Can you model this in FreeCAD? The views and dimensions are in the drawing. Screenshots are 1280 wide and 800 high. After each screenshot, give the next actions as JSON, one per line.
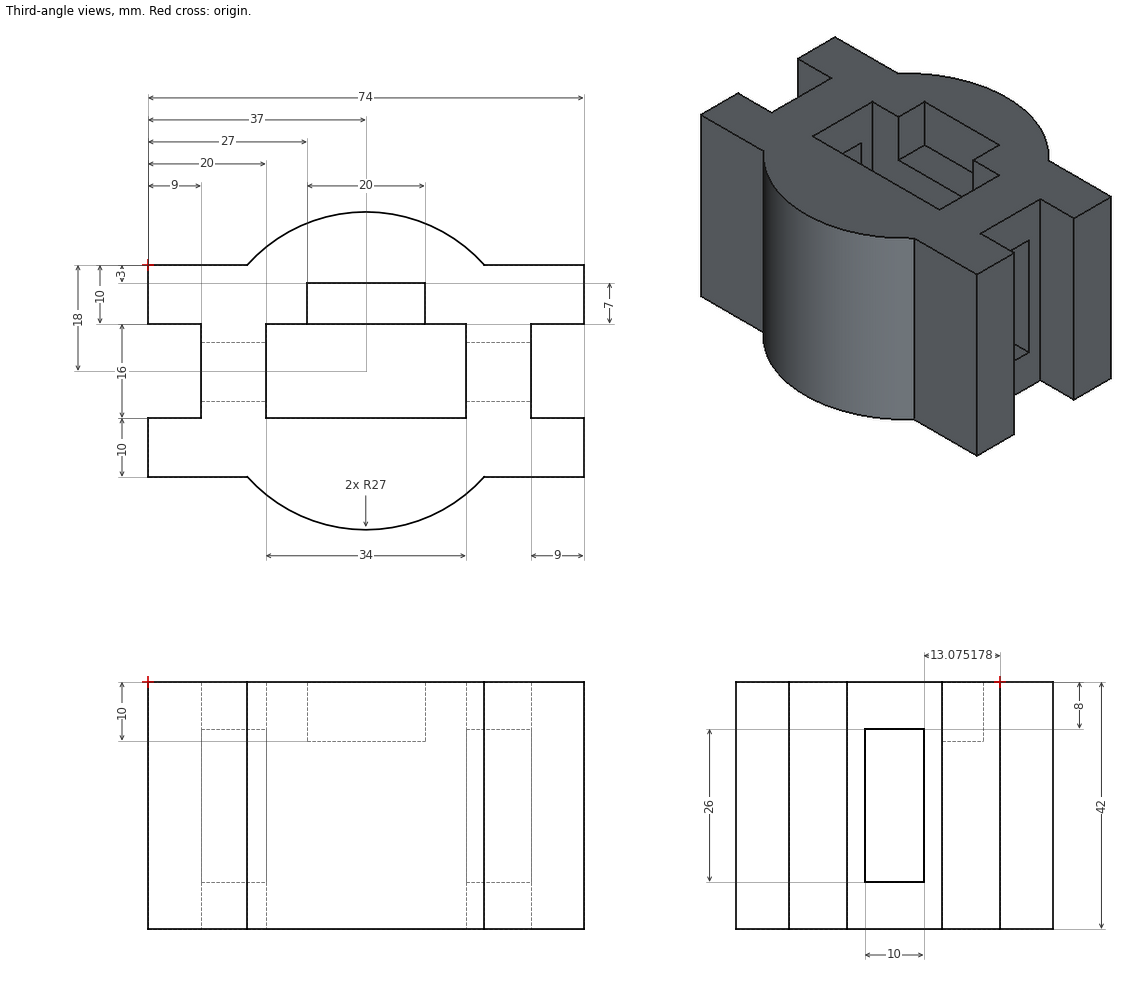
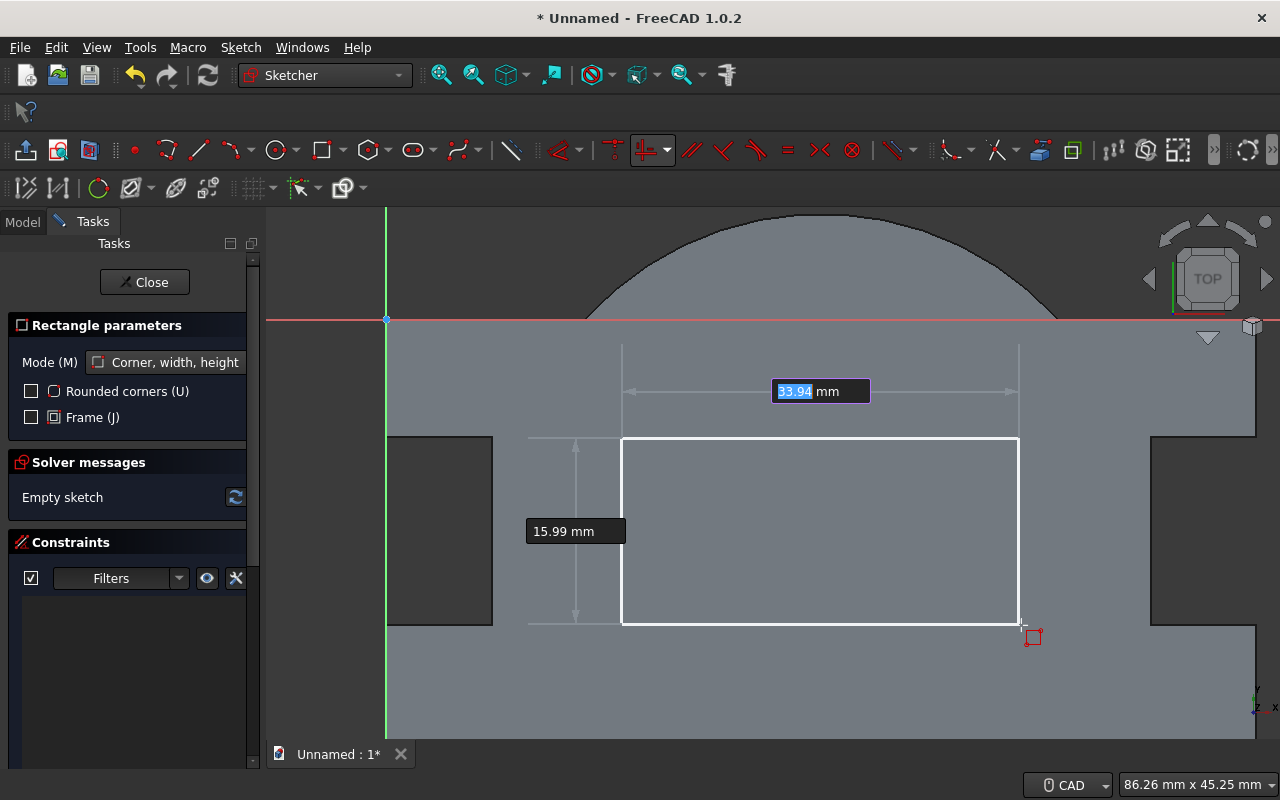
{"action": "type", "text": "34"}
{"action": "key", "text": "Tab"}
{"action": "type", "text": "16"}
{"action": "key", "text": "Return"}
{"action": "key", "text": "Escape"}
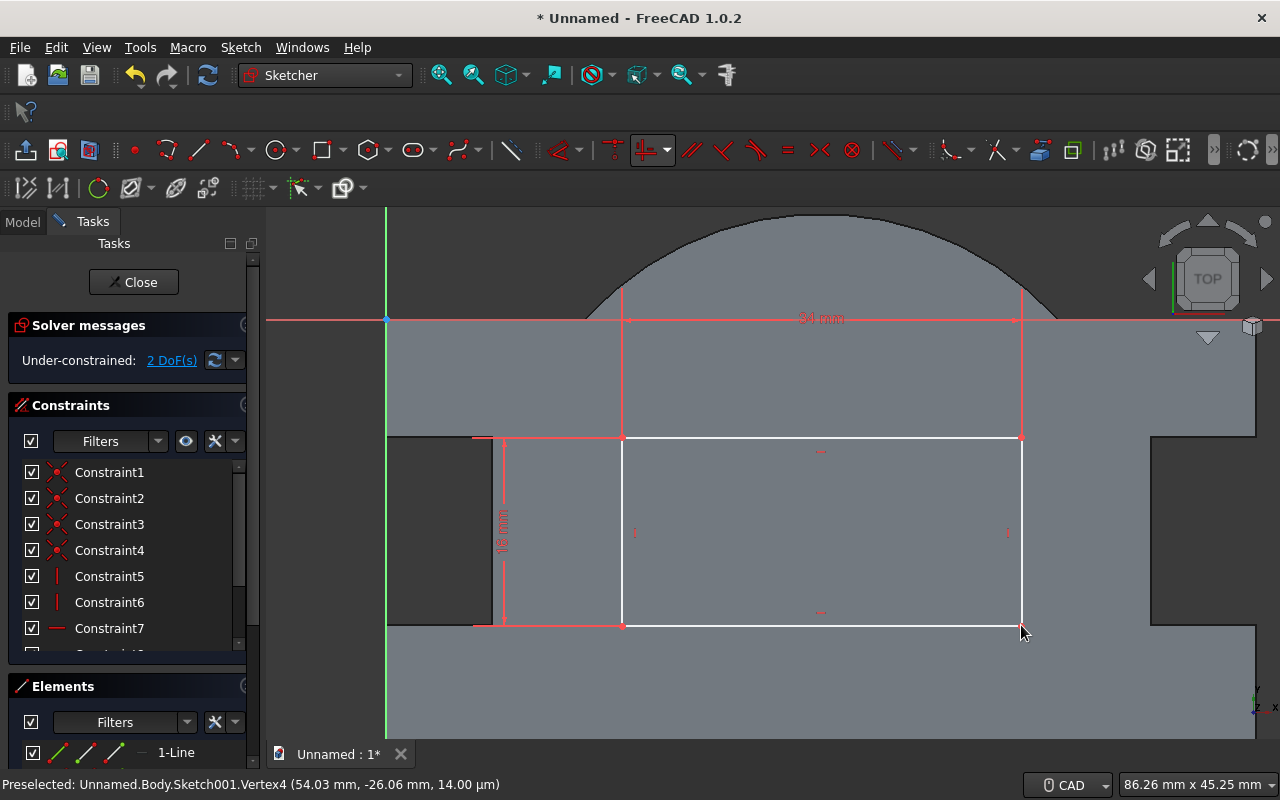
{"action": "left_click", "coordinate": [558, 150]}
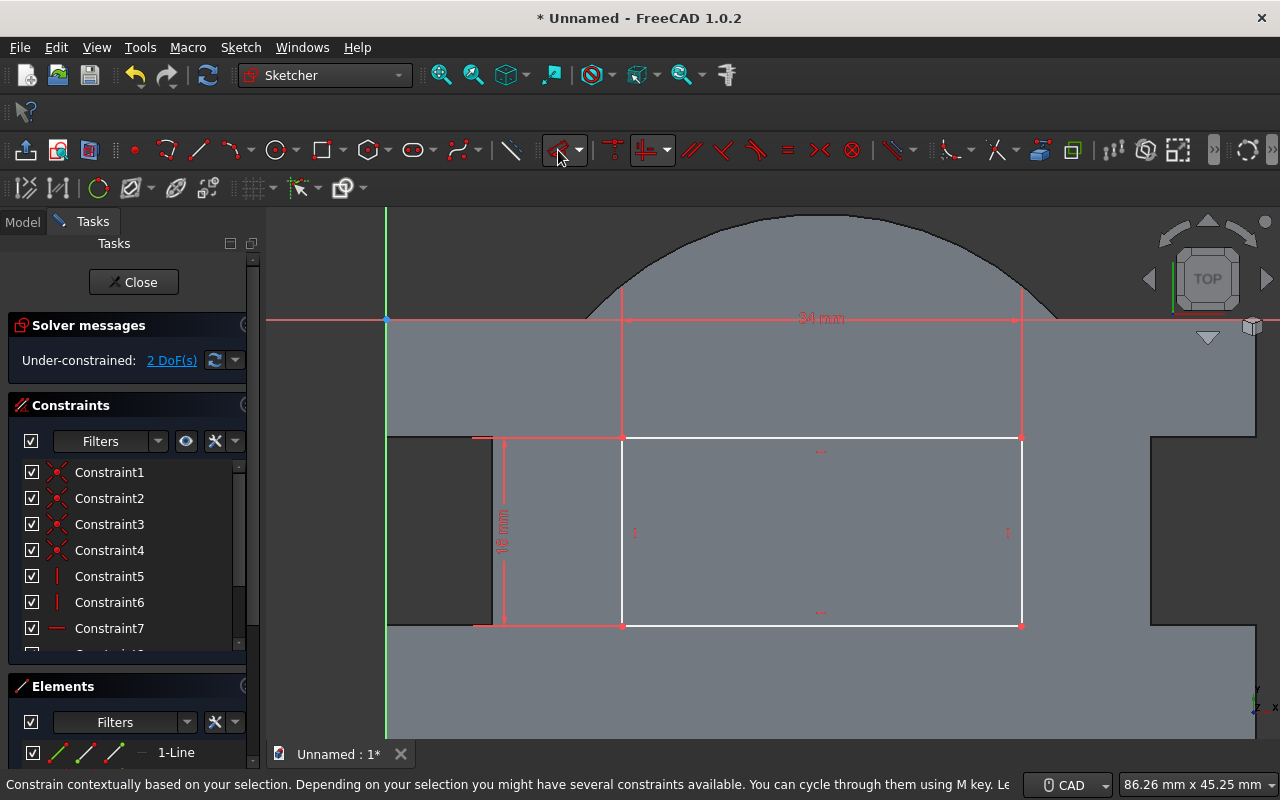
{"action": "left_click", "coordinate": [622, 438]}
{"action": "left_click", "coordinate": [504, 286]}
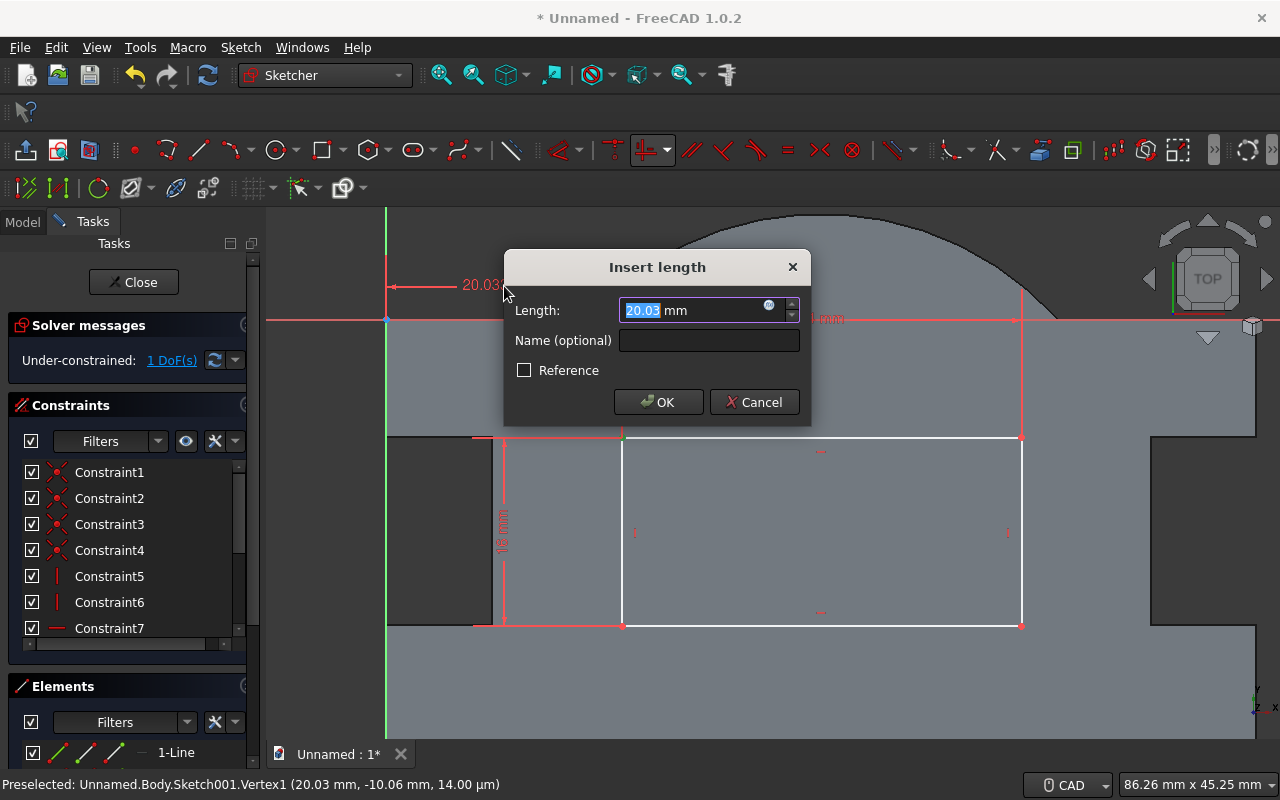
{"action": "type", "text": "20"}
{"action": "key", "text": "Return"}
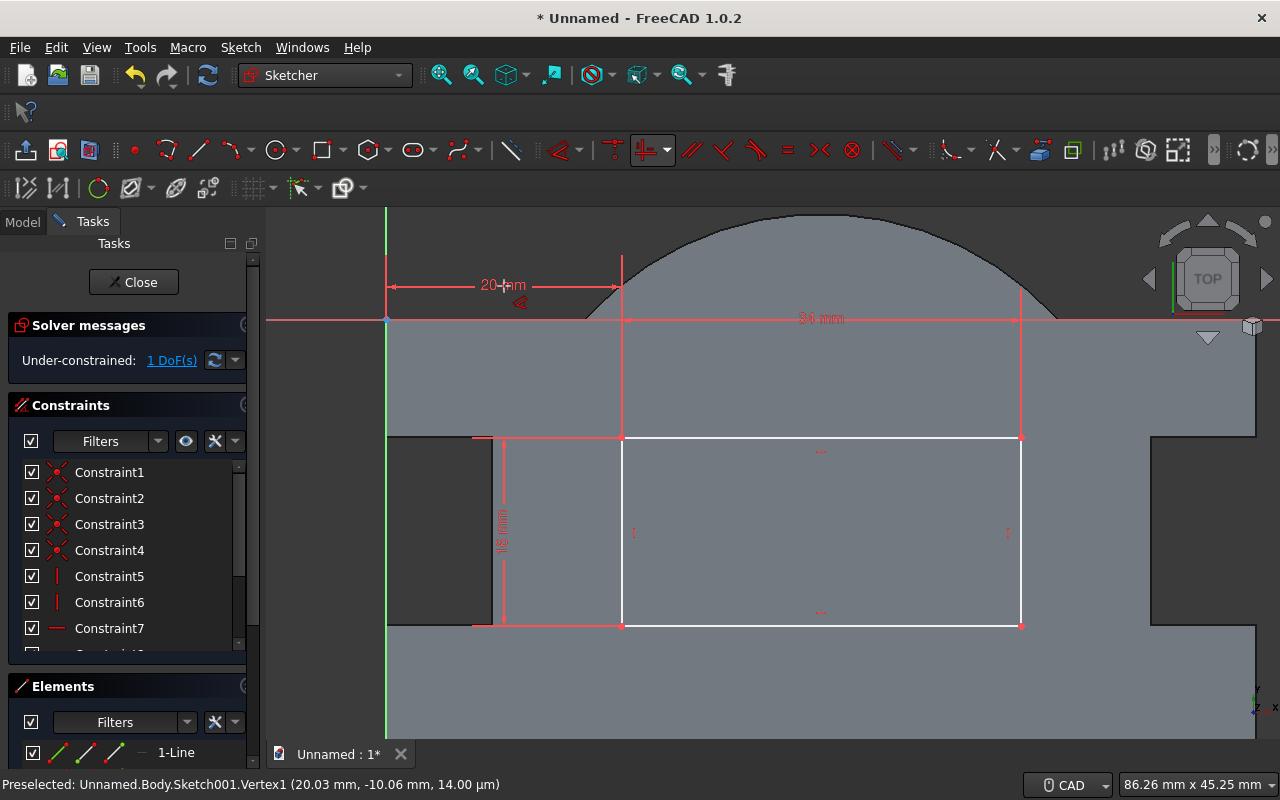
{"action": "left_click", "coordinate": [622, 438]}
{"action": "left_click", "coordinate": [352, 379]}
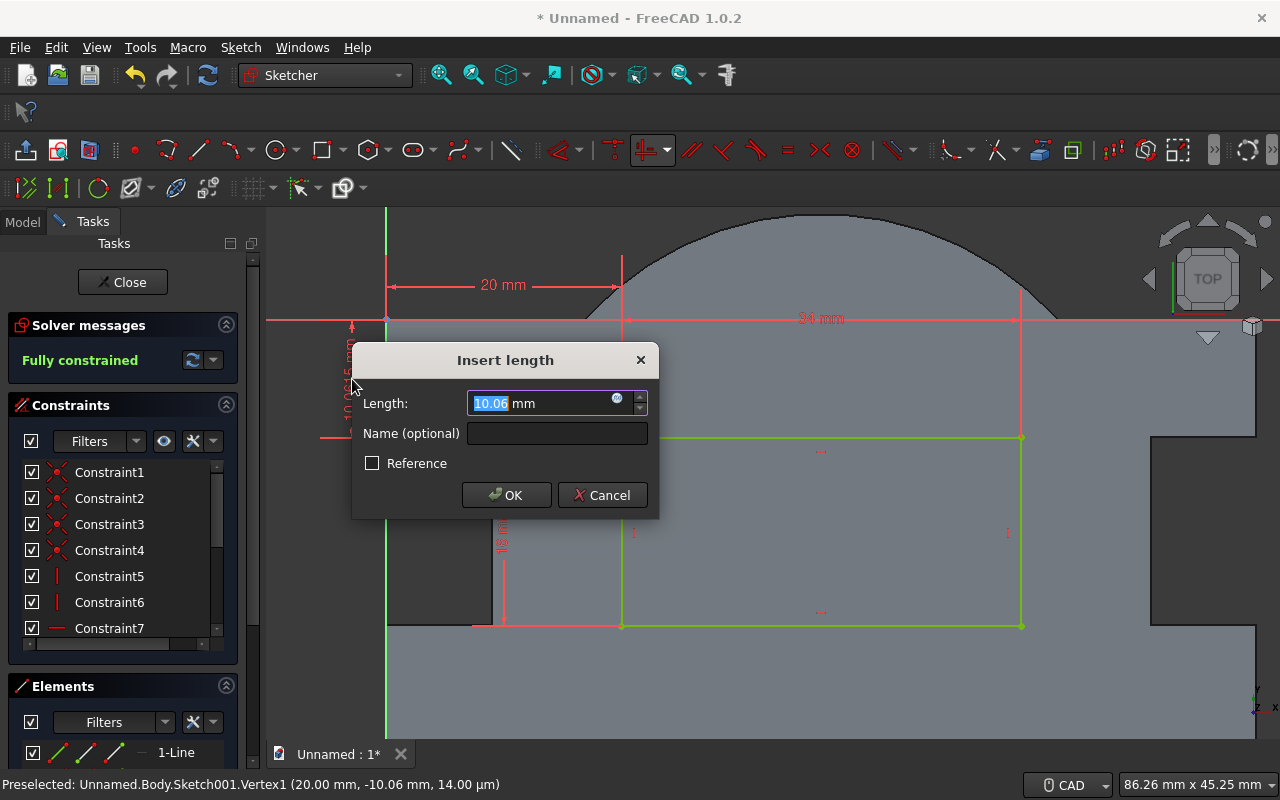
{"action": "type", "text": "10"}
{"action": "key", "text": "Return"}
{"action": "key", "text": "Escape"}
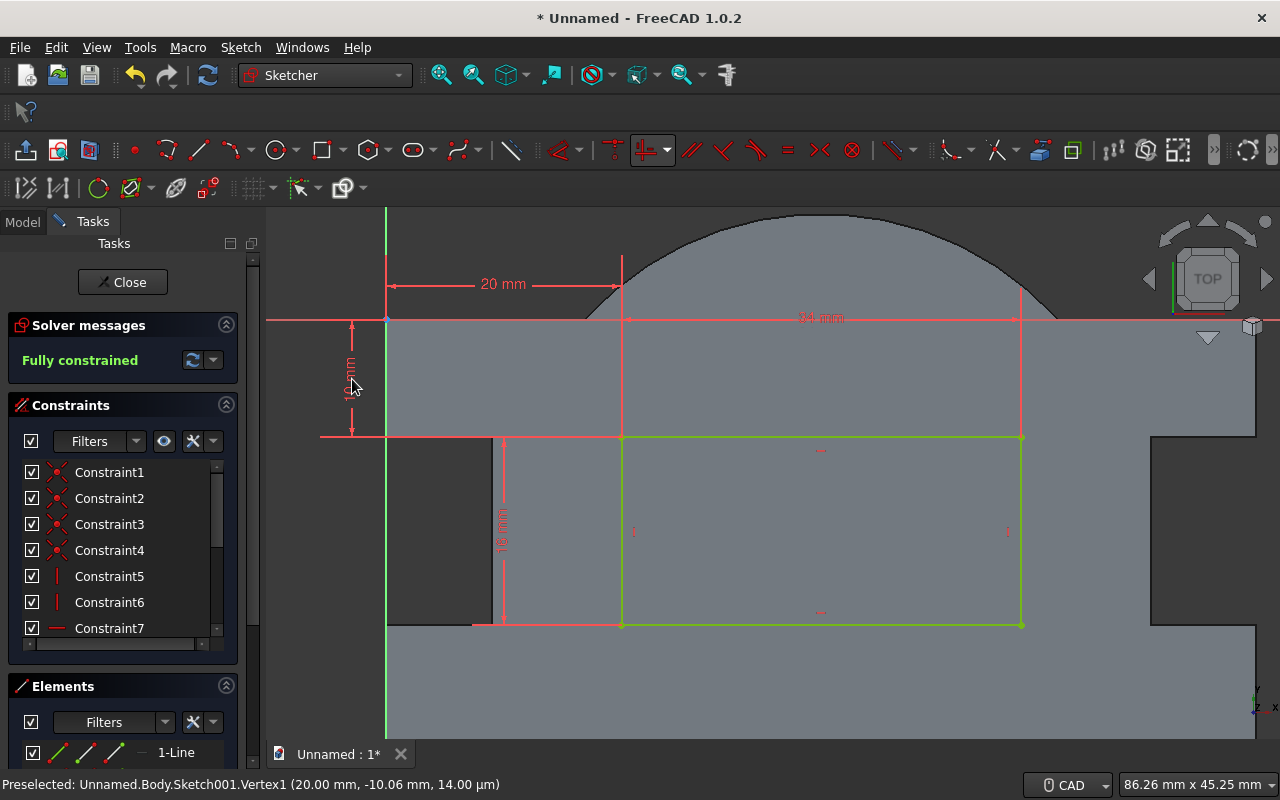
{"action": "left_click", "coordinate": [123, 282]}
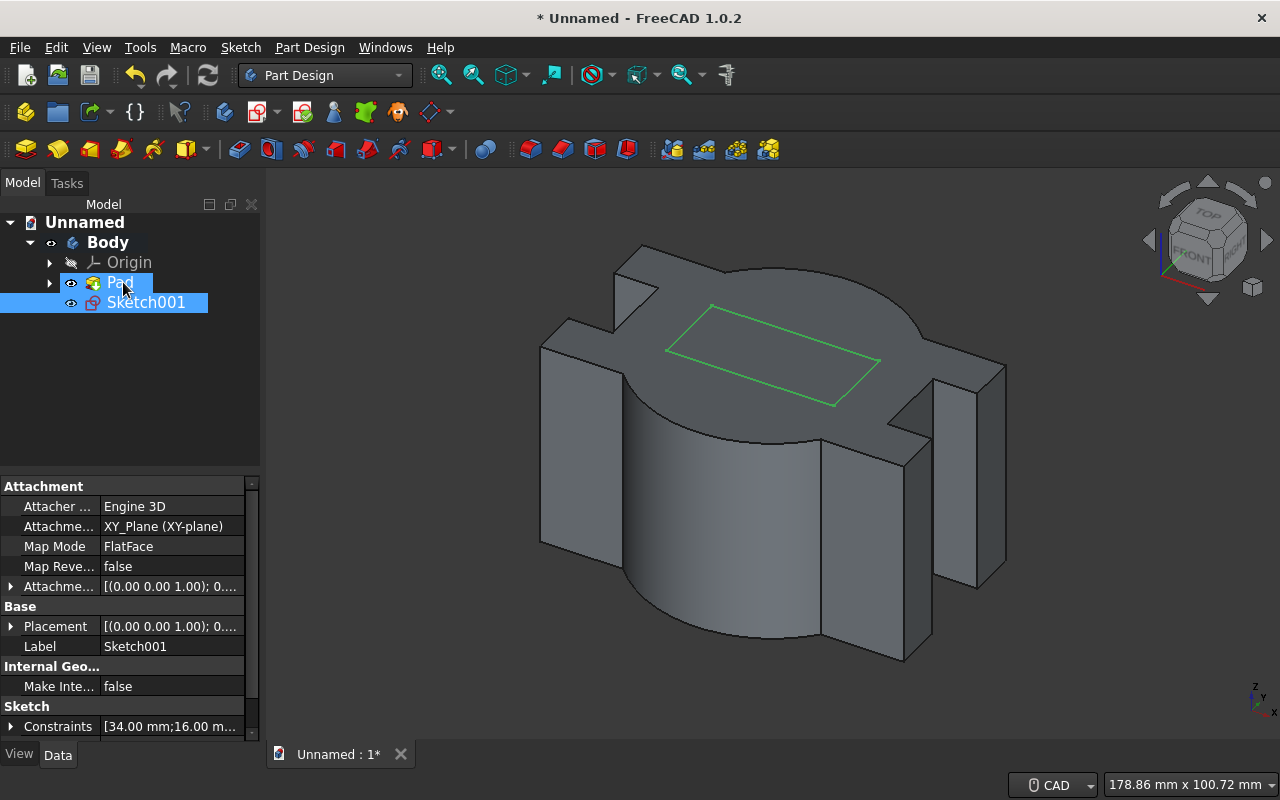
{"action": "left_click", "coordinate": [240, 150]}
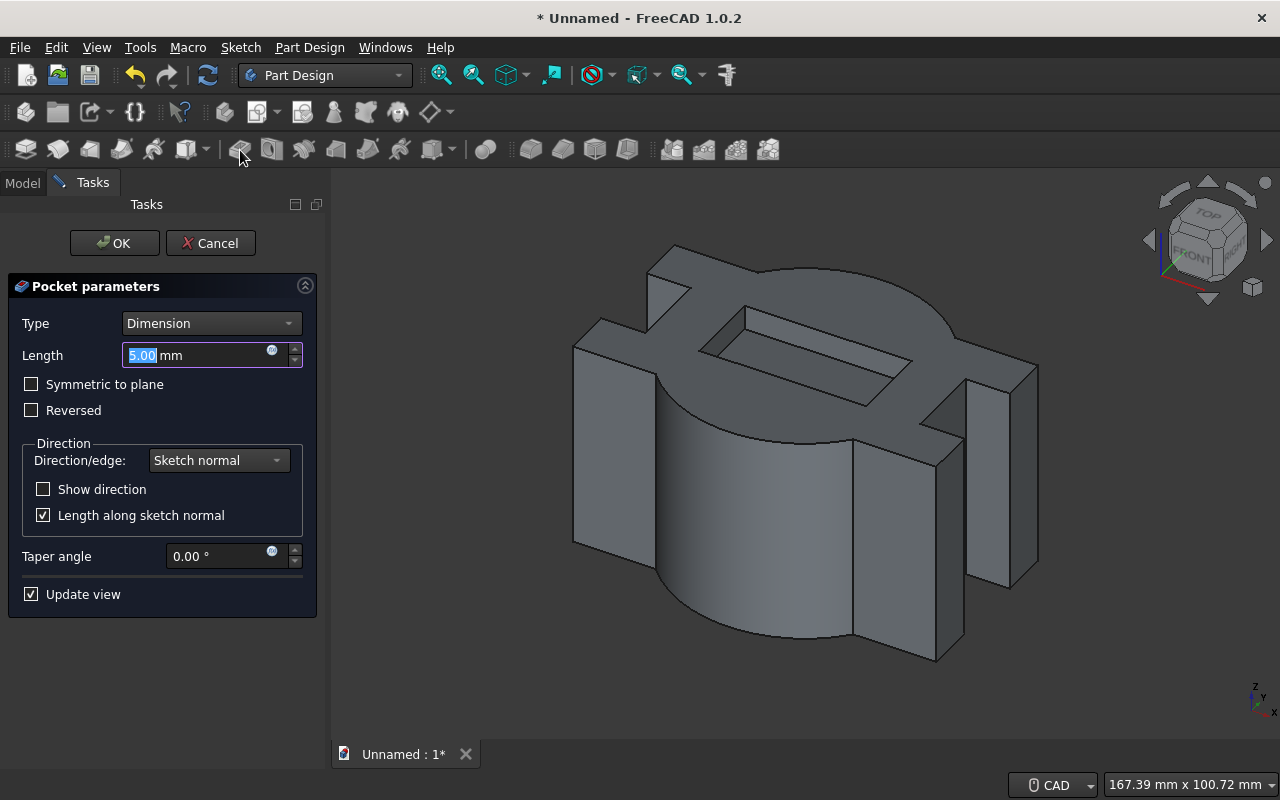
{"action": "left_click", "coordinate": [212, 324]}